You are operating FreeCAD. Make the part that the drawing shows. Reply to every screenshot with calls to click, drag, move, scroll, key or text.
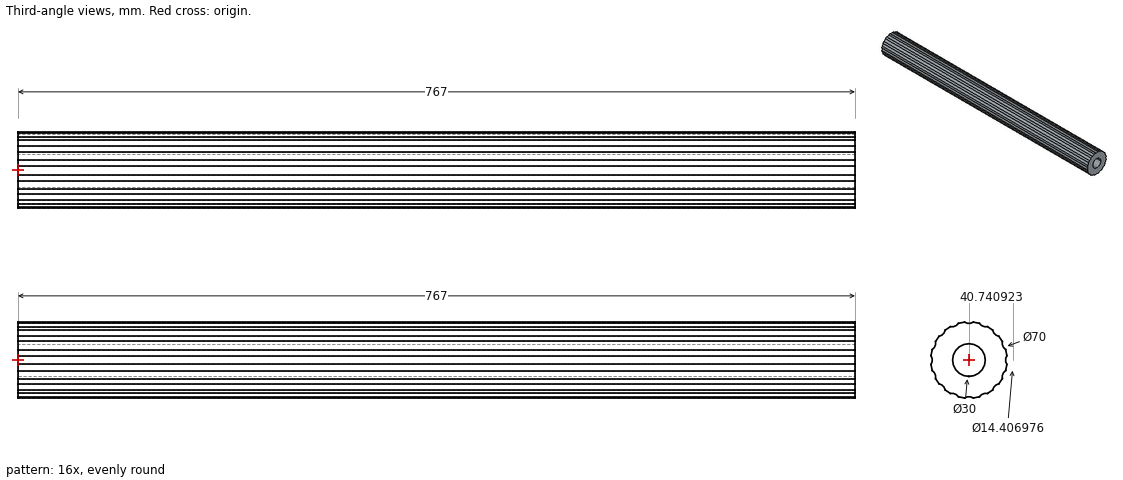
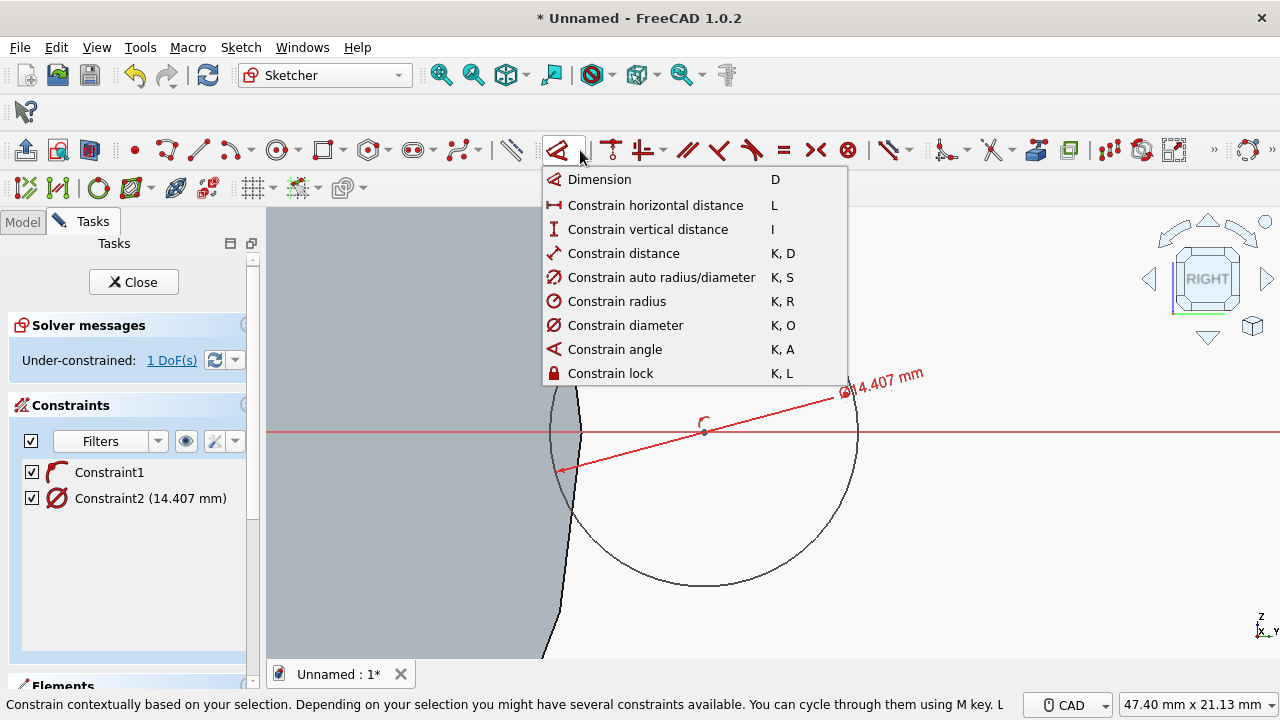
click(695, 205)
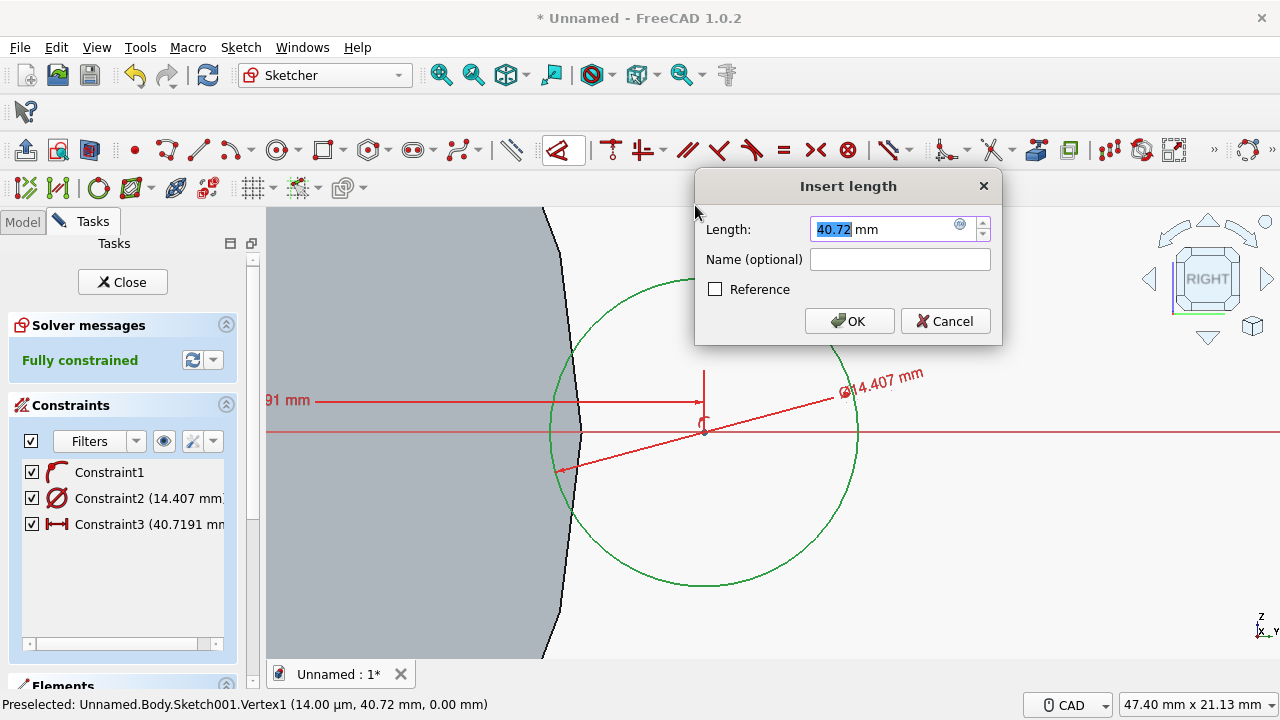
text(40.740923)
key(Return)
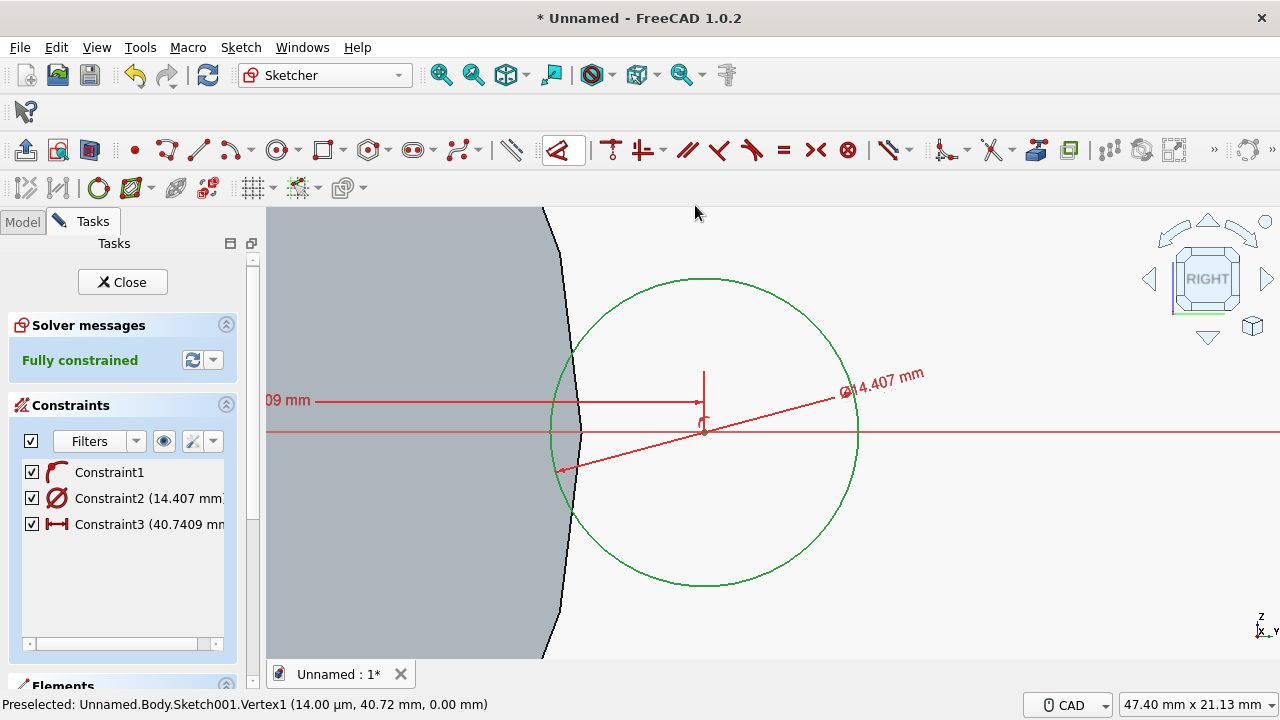
click(123, 282)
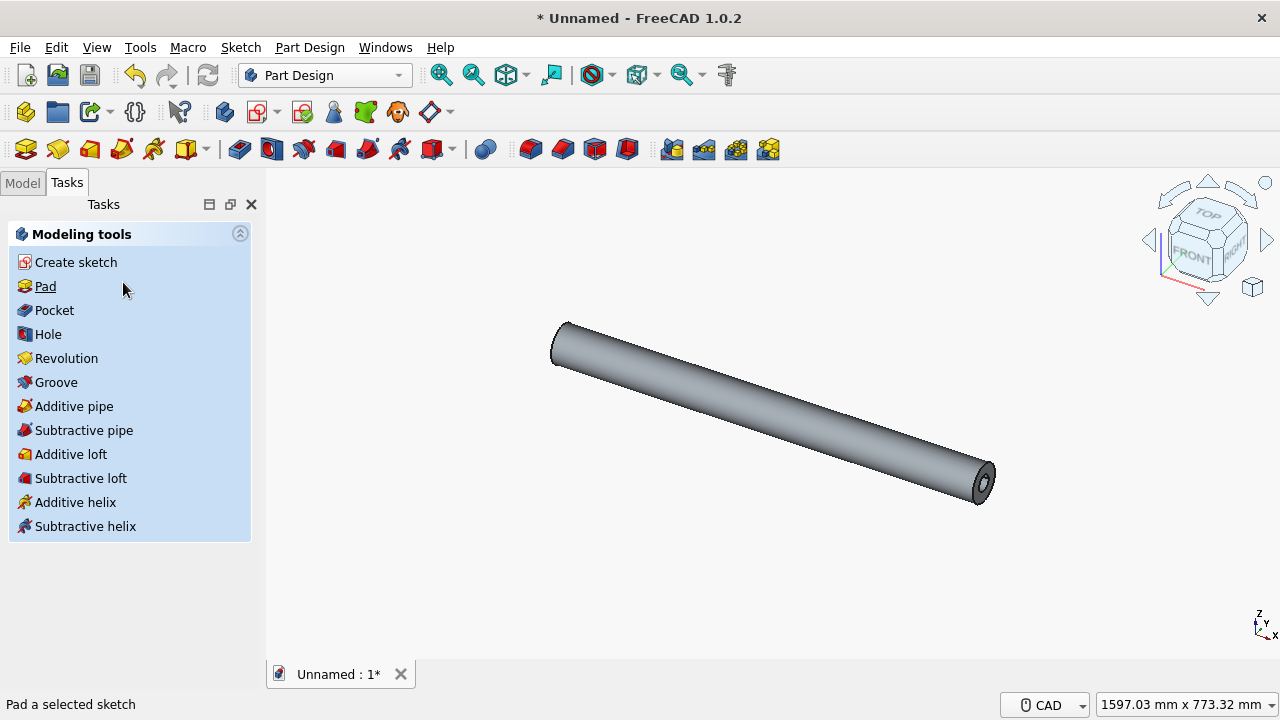
click(240, 150)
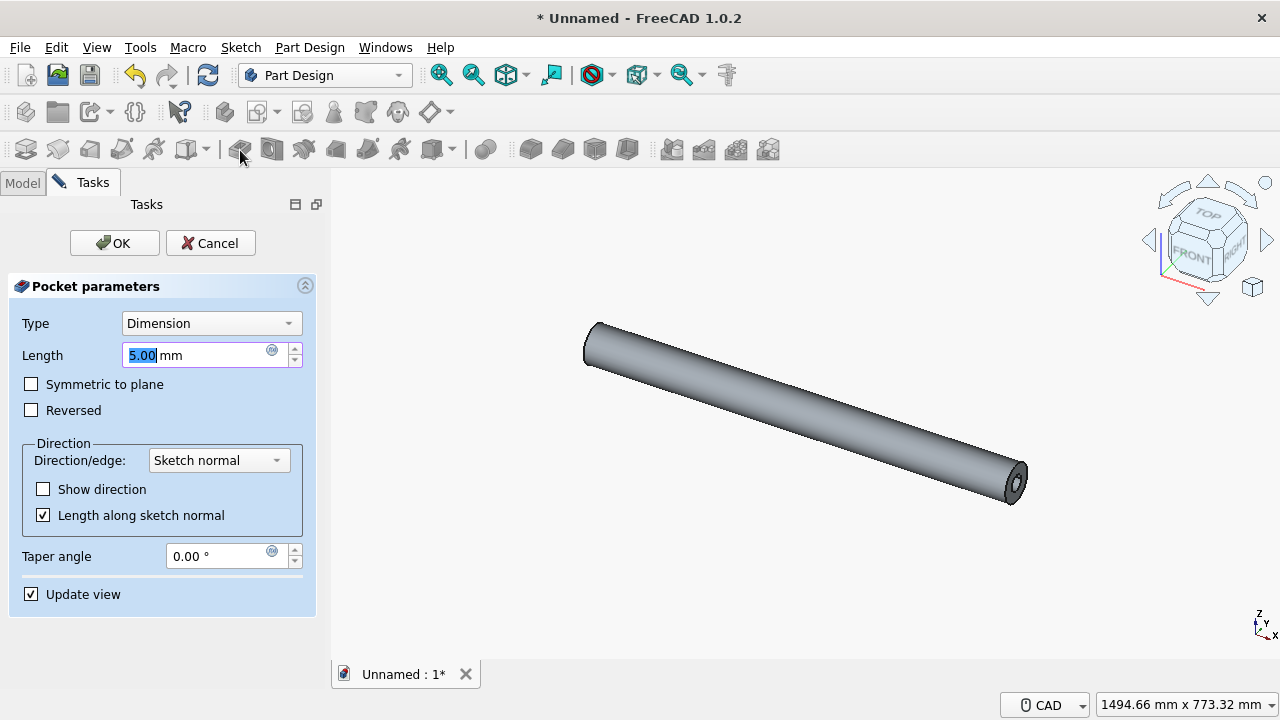
text(767)
key(Tab)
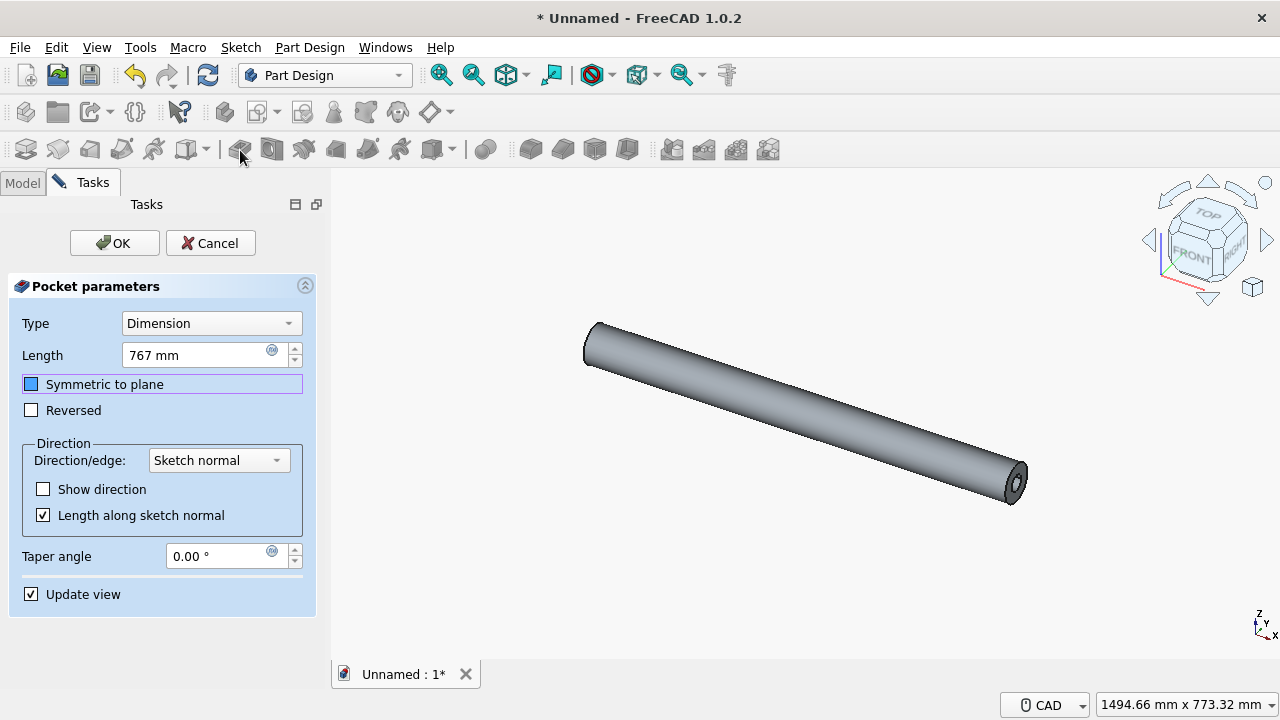
click(30, 410)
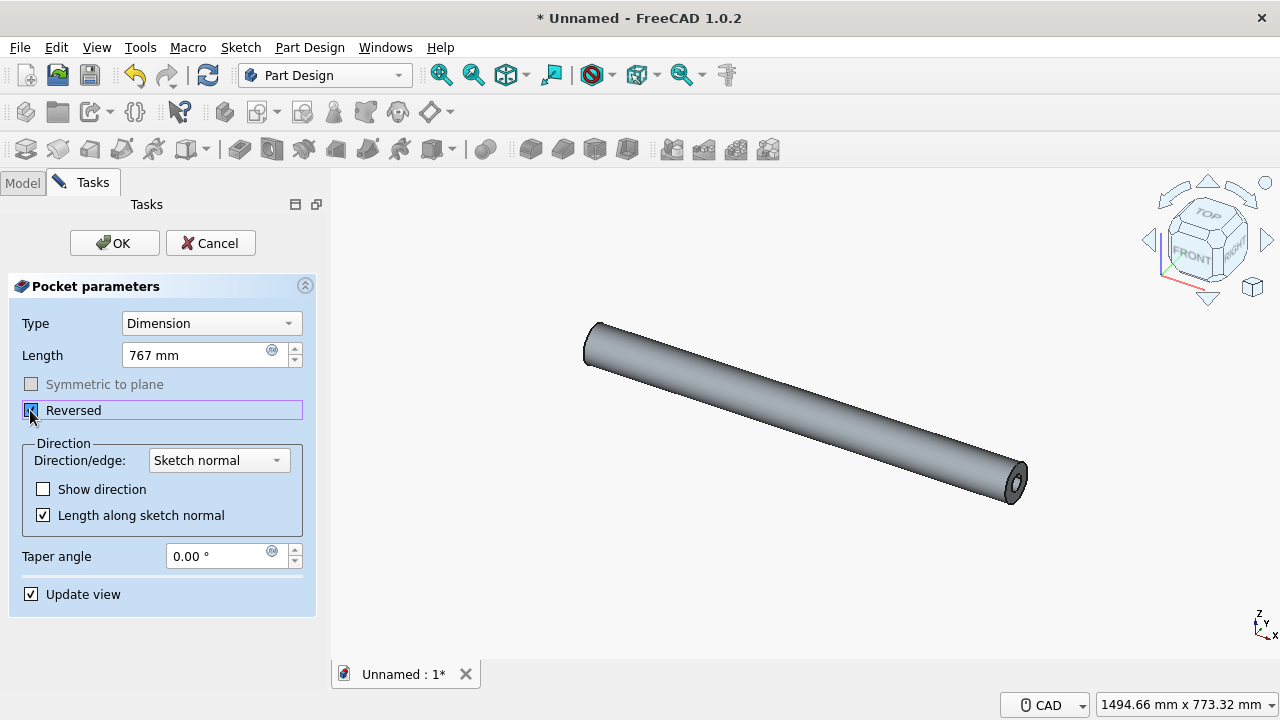
click(115, 243)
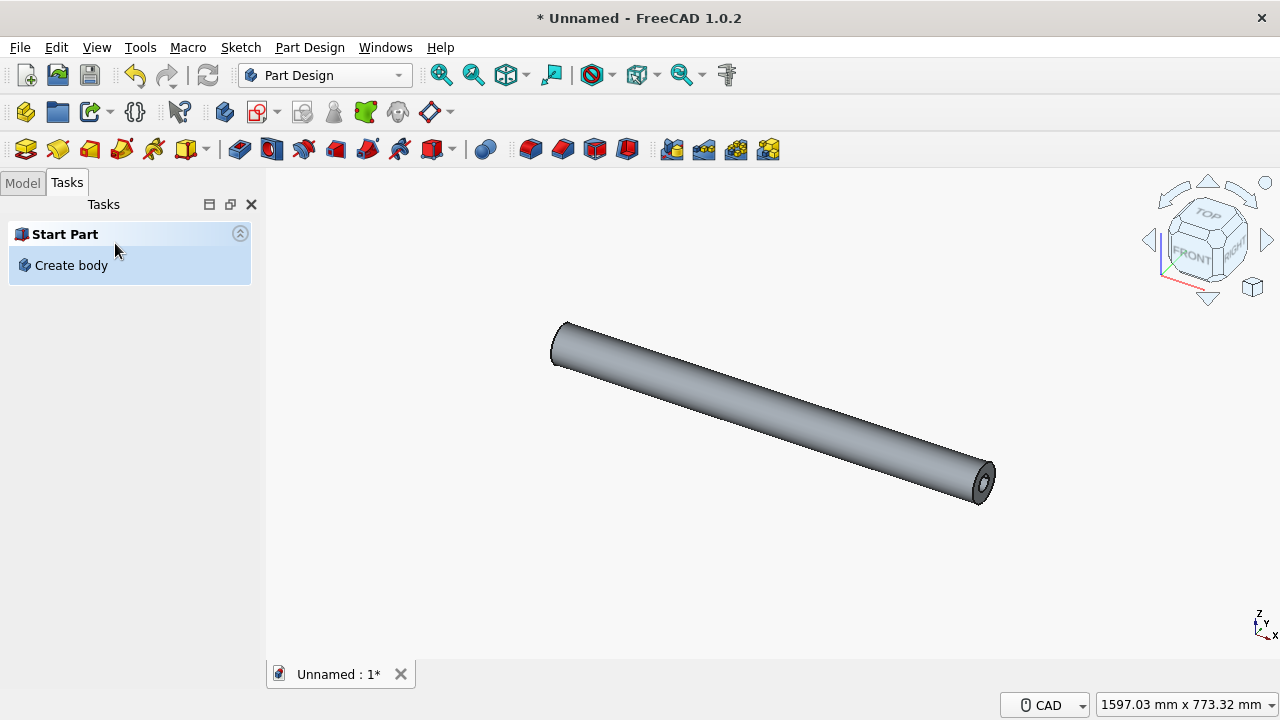
click(442, 76)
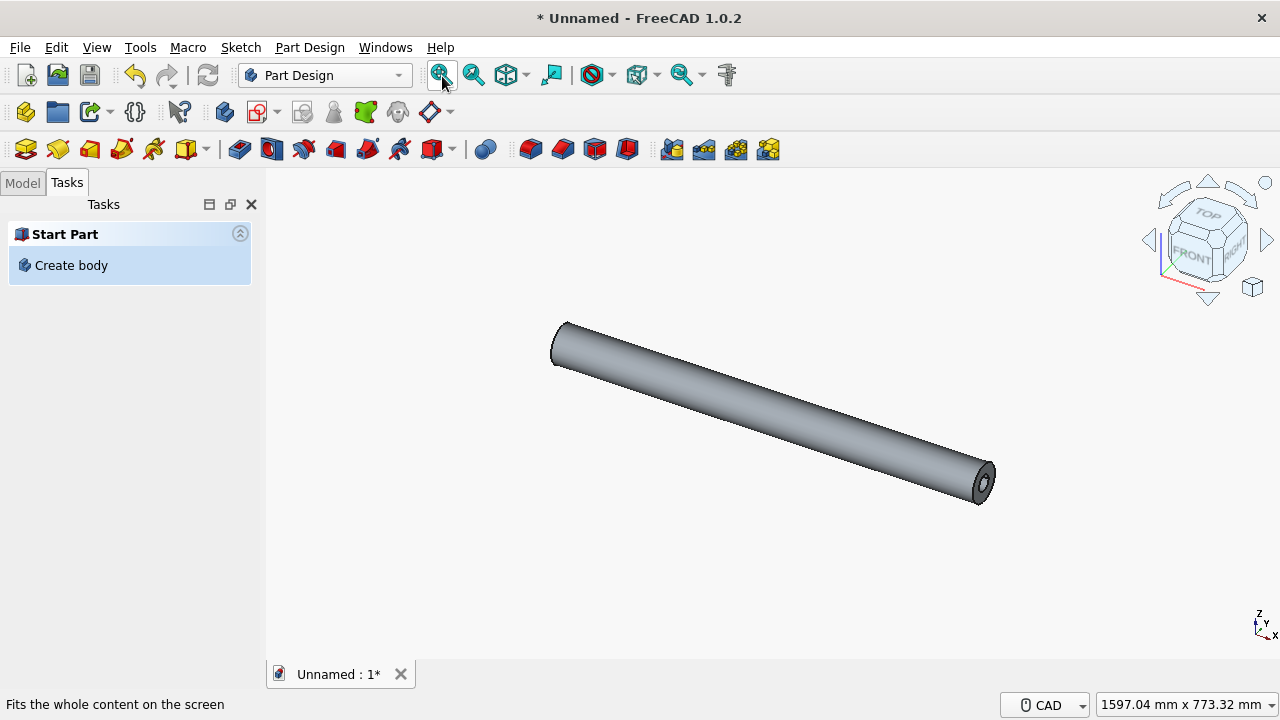
click(23, 182)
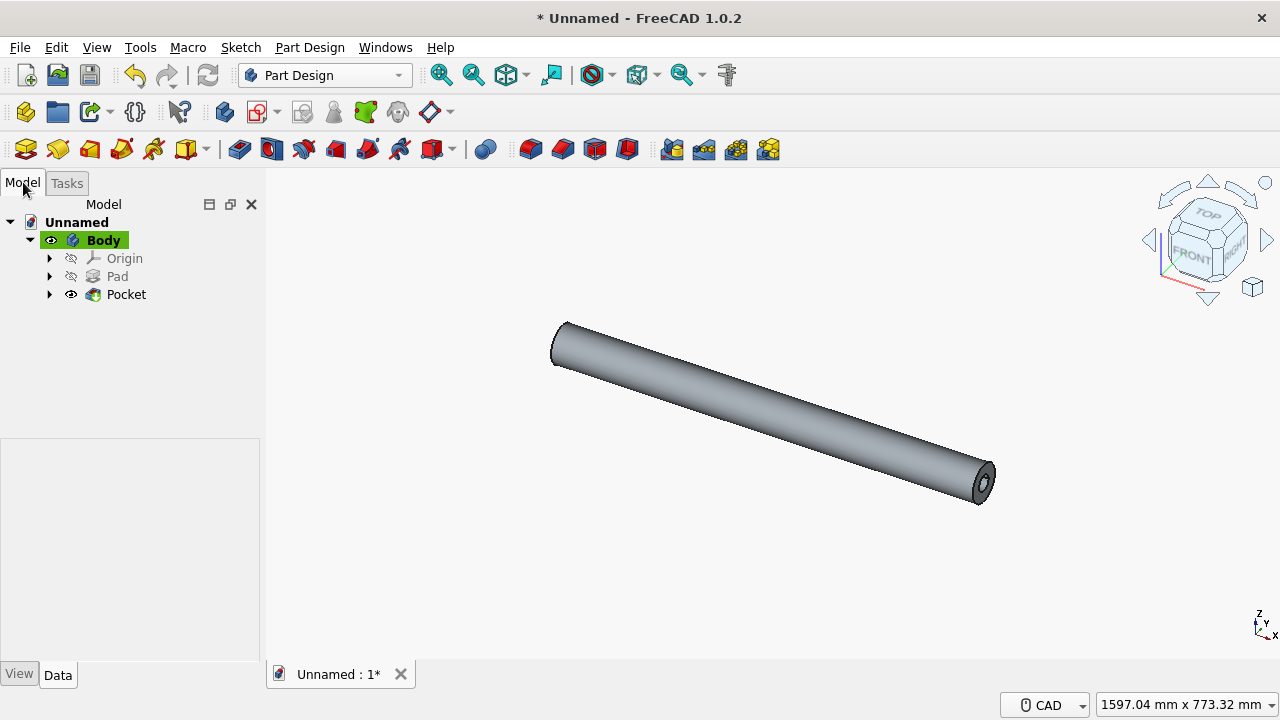
click(116, 294)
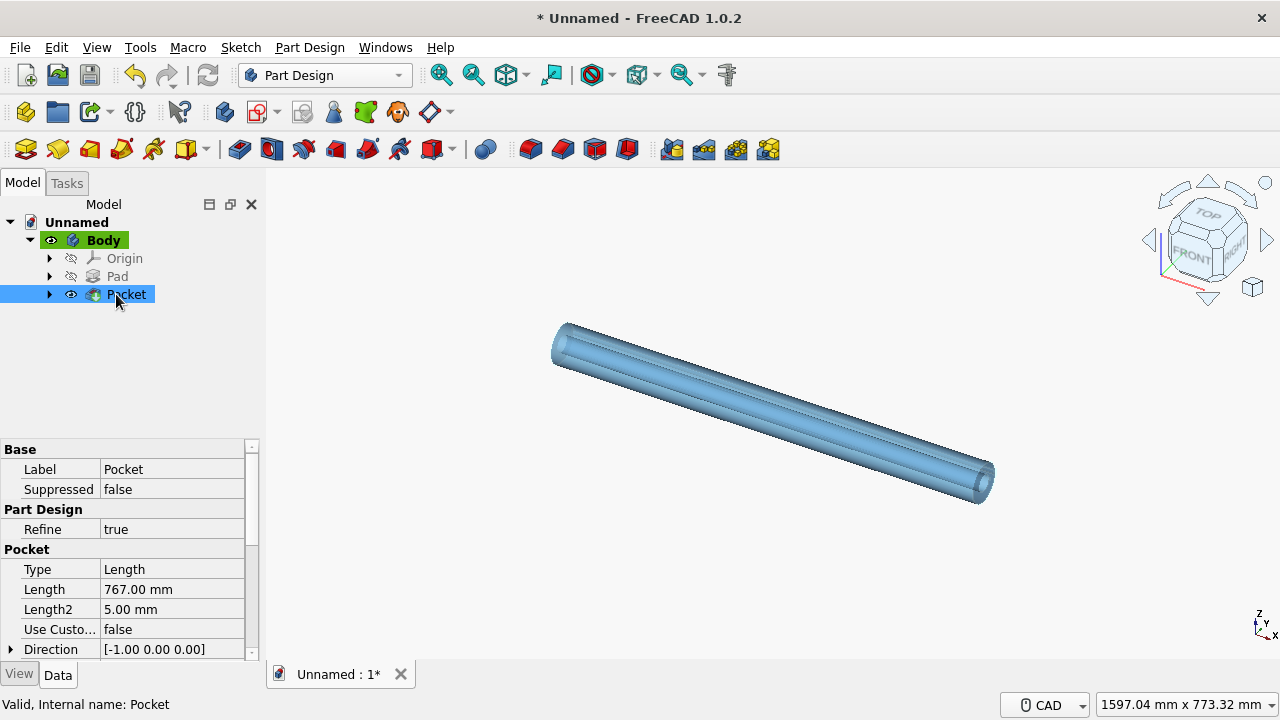
click(736, 150)